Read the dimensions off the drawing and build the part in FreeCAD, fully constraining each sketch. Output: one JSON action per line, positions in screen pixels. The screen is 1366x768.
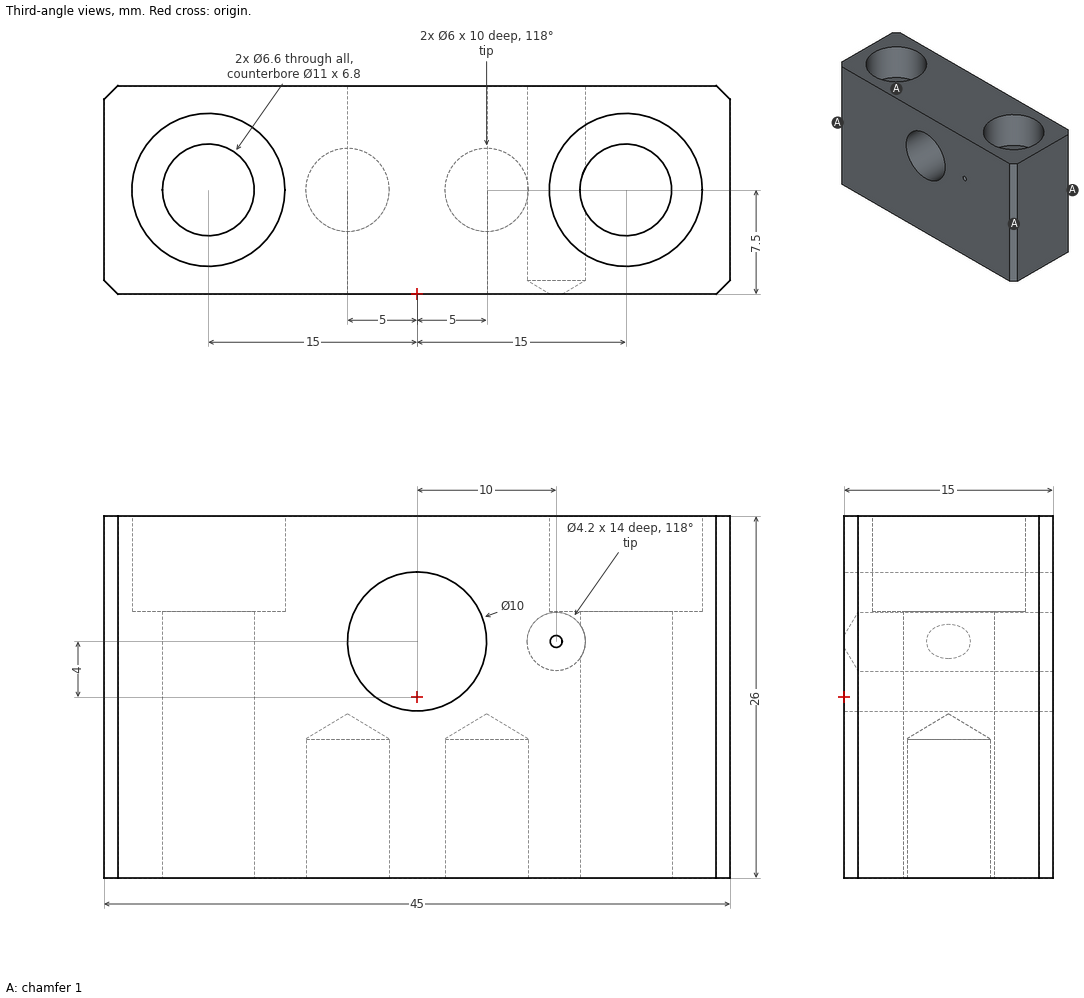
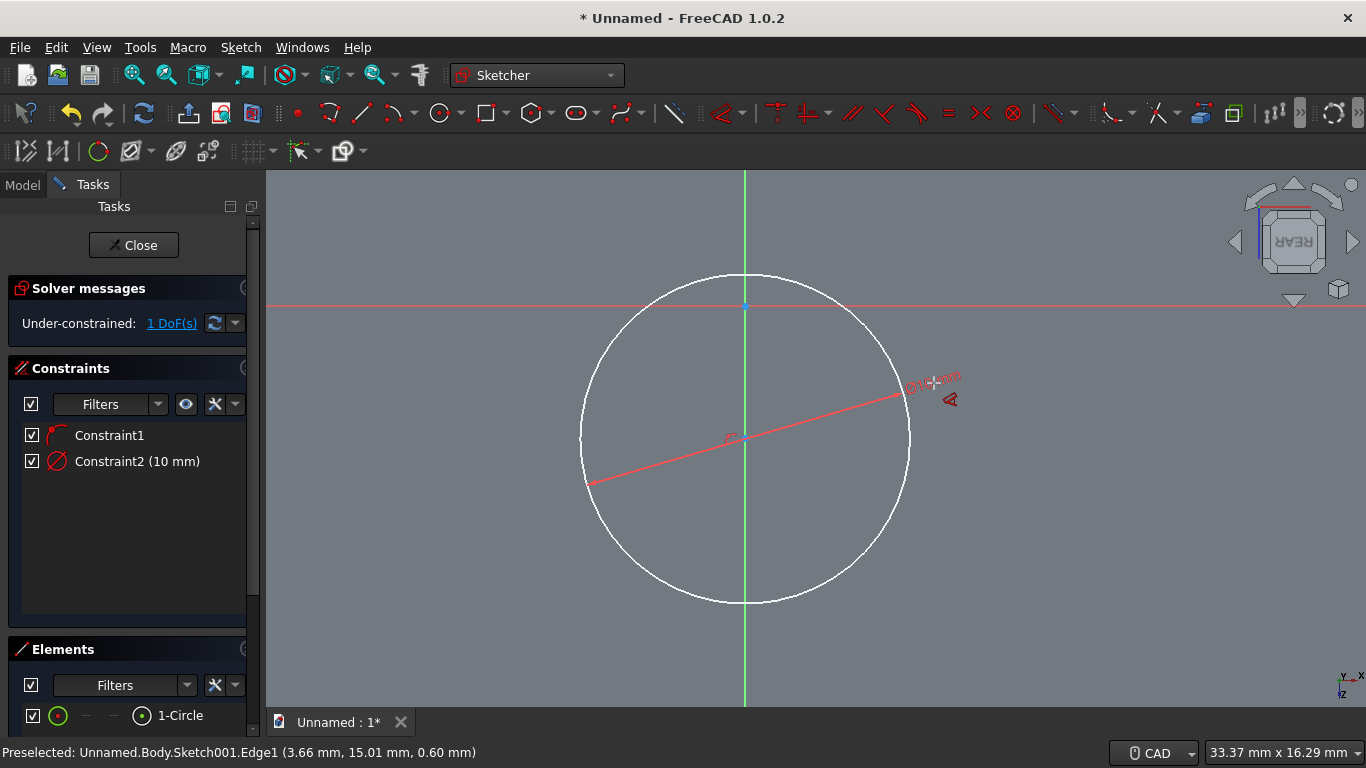
{"action": "left_click", "coordinate": [745, 439]}
{"action": "left_click", "coordinate": [779, 373]}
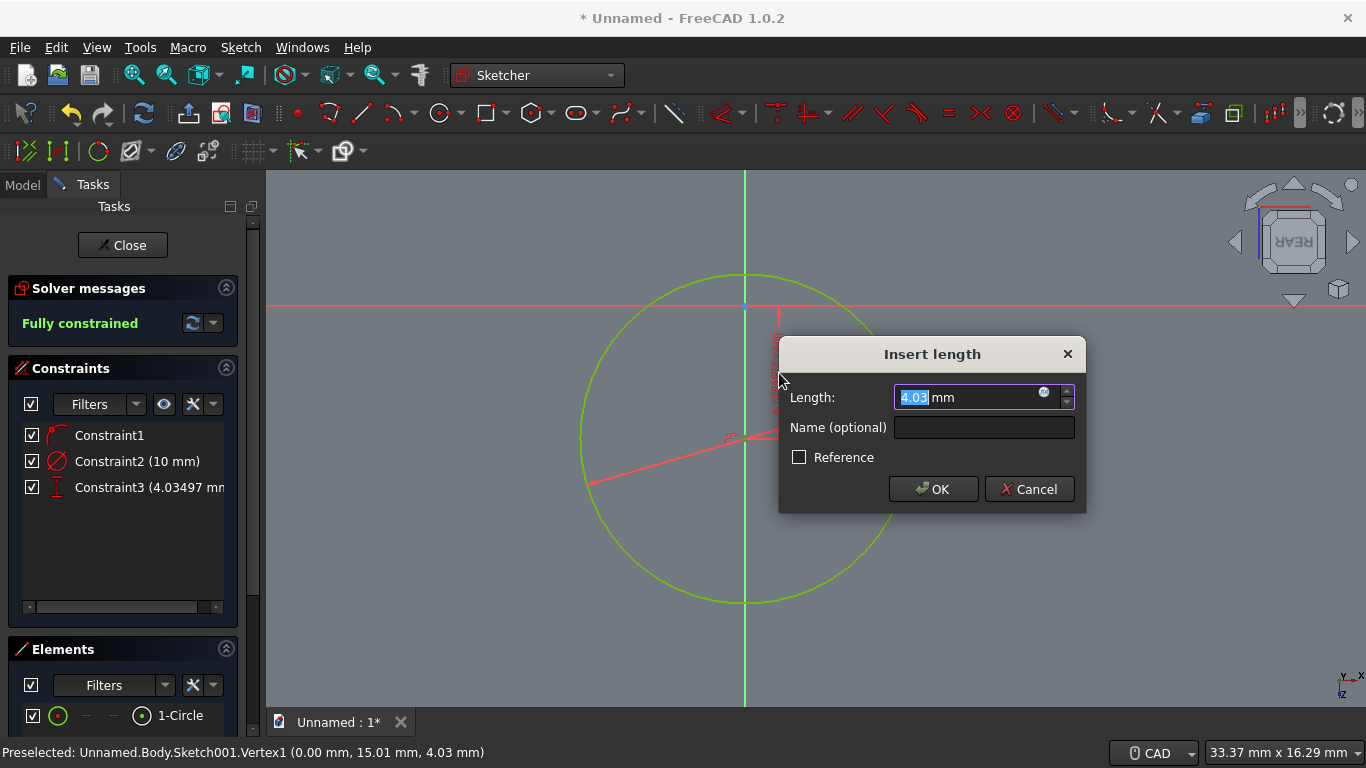
{"action": "type", "text": "4"}
{"action": "key", "text": "Return"}
{"action": "key", "text": "Escape"}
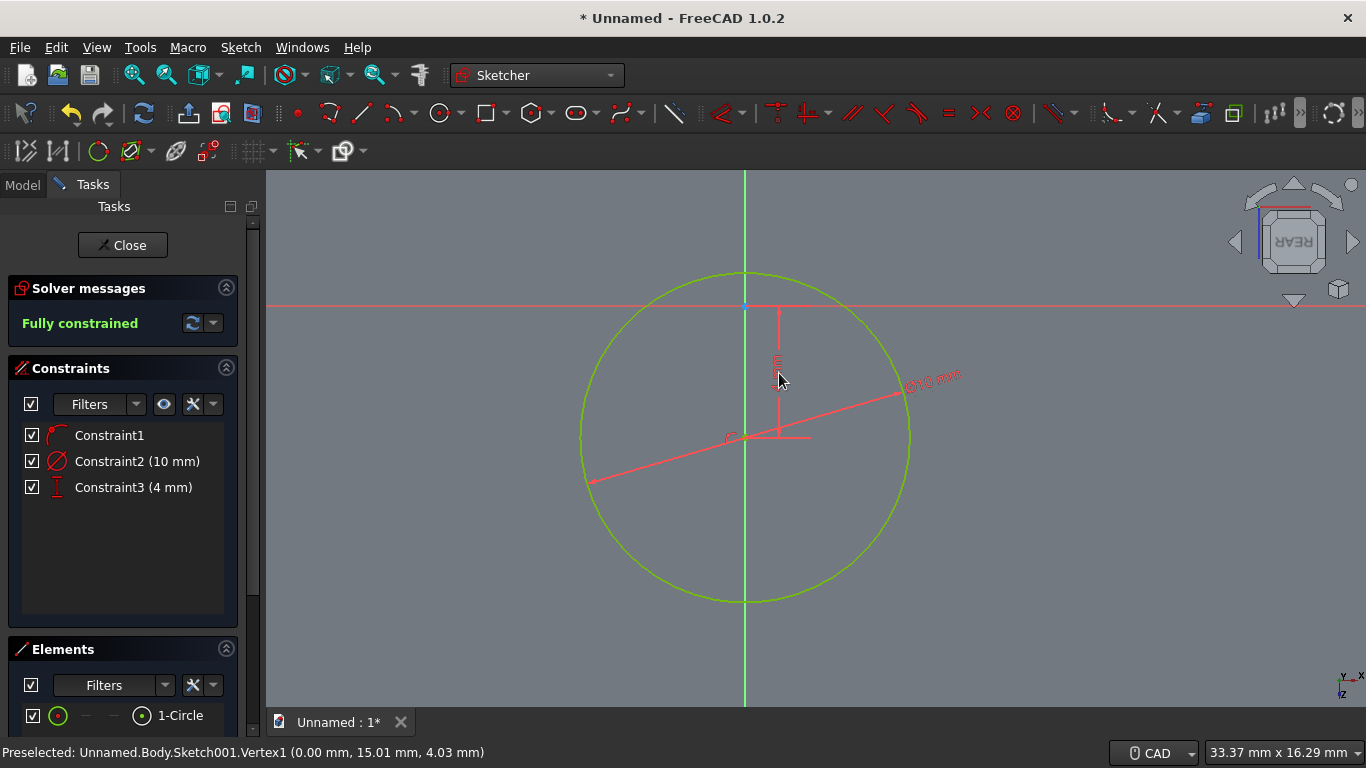
{"action": "left_click", "coordinate": [123, 245]}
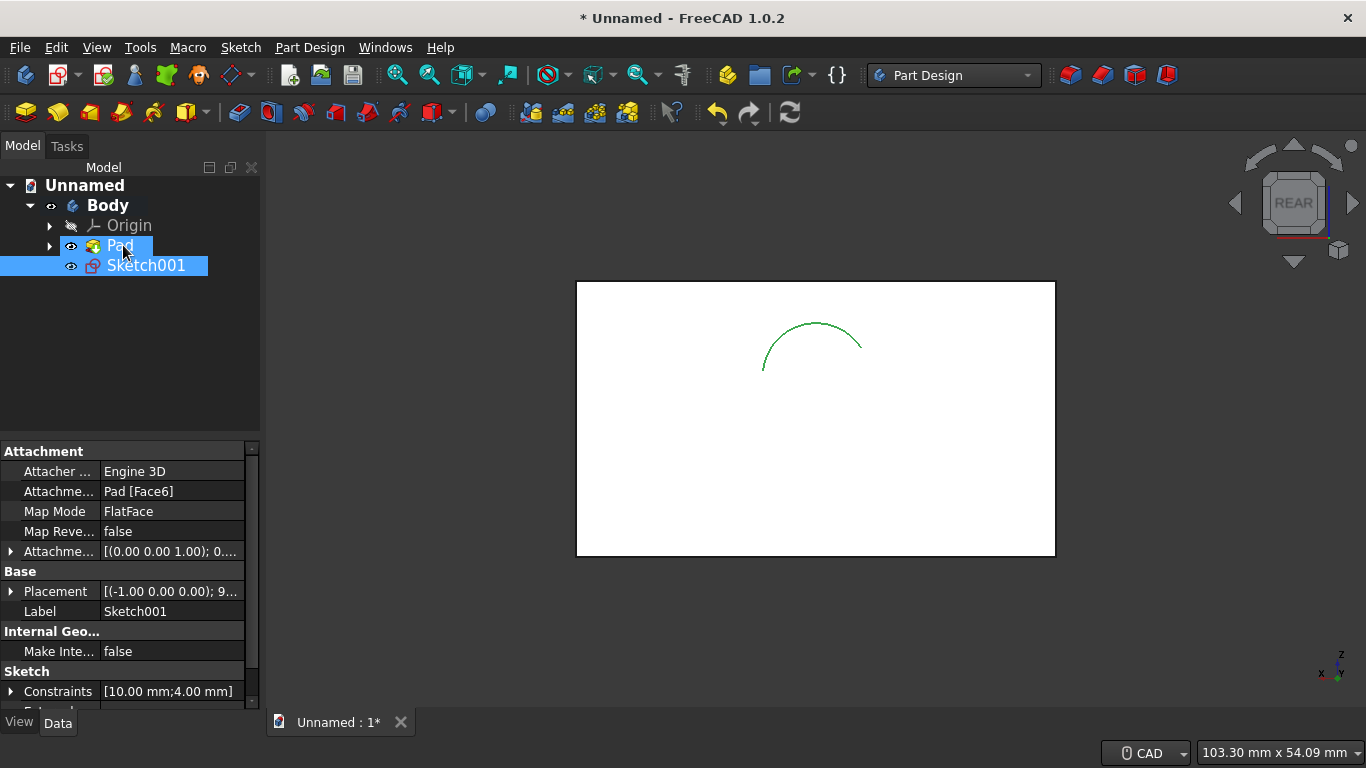
{"action": "left_click", "coordinate": [240, 112]}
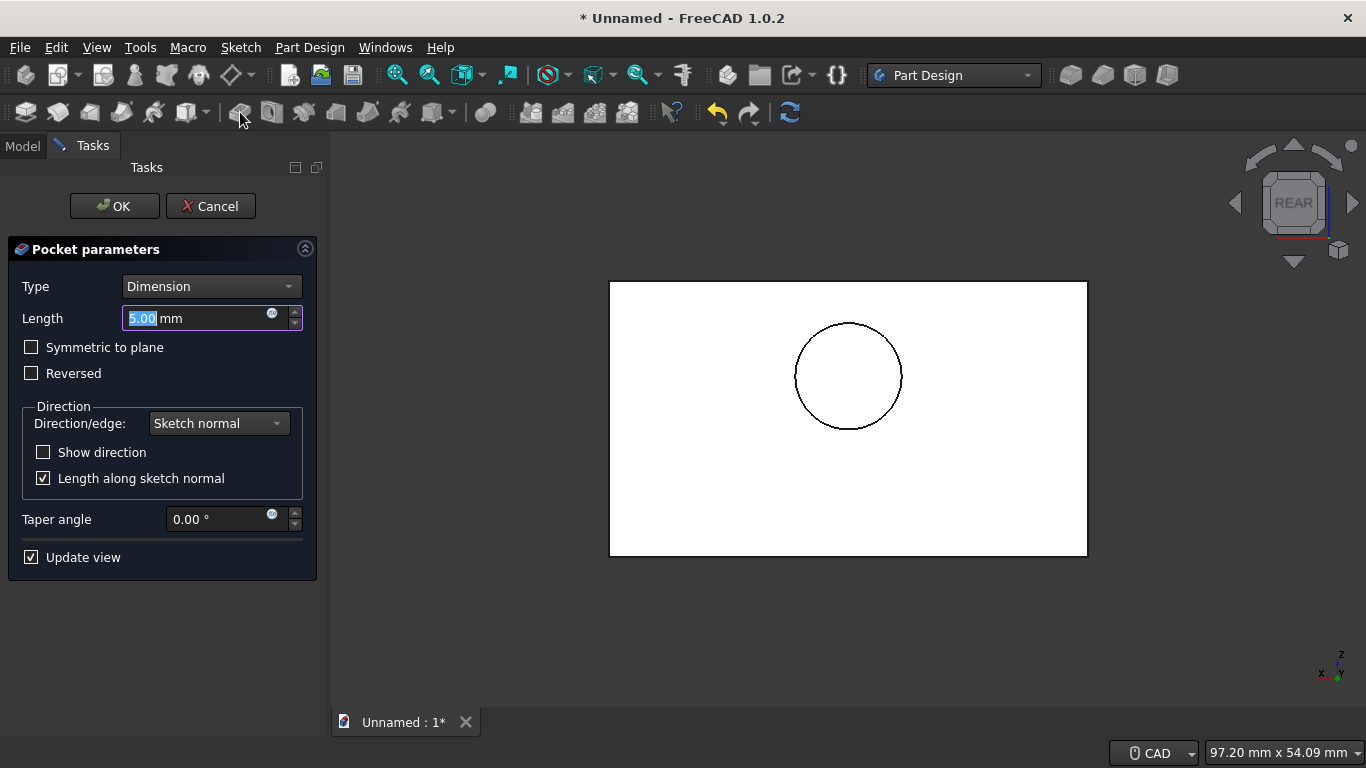
{"action": "left_click", "coordinate": [212, 286]}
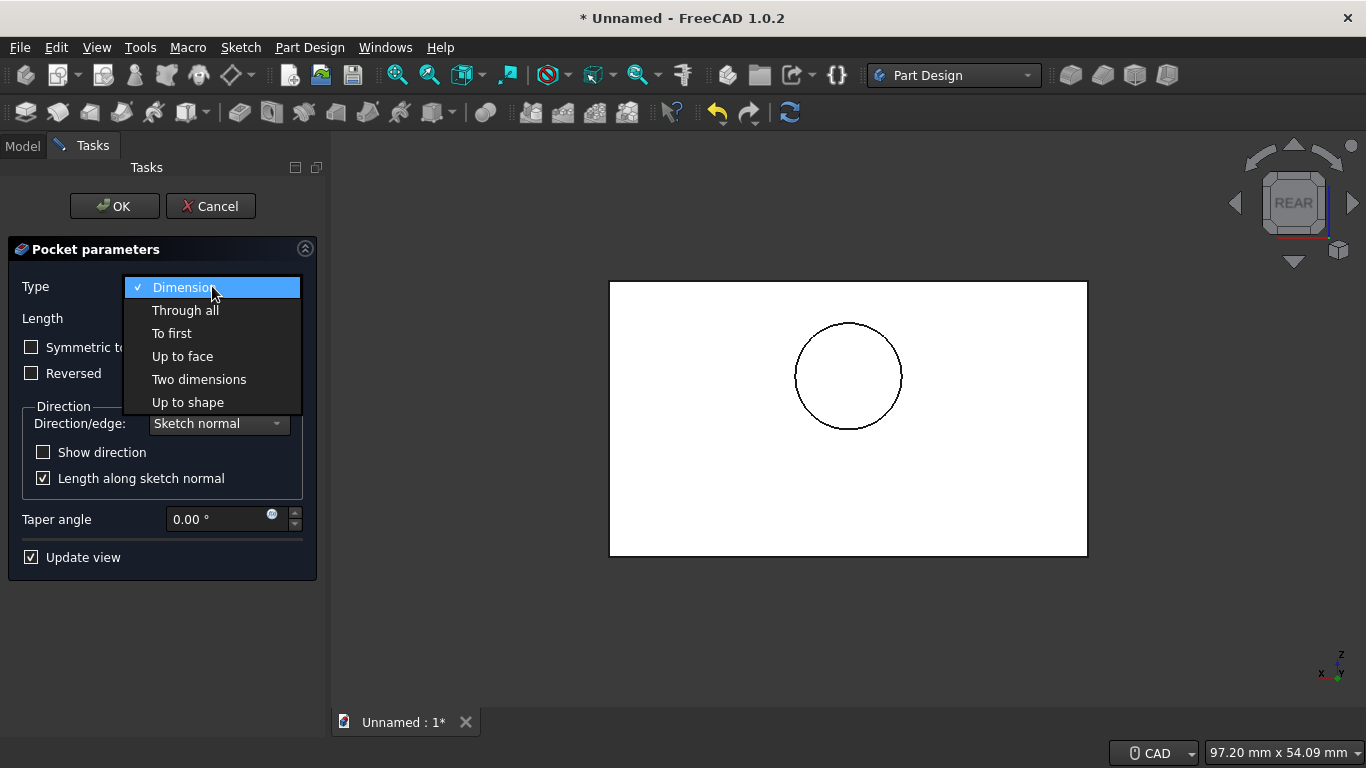
{"action": "left_click", "coordinate": [212, 310]}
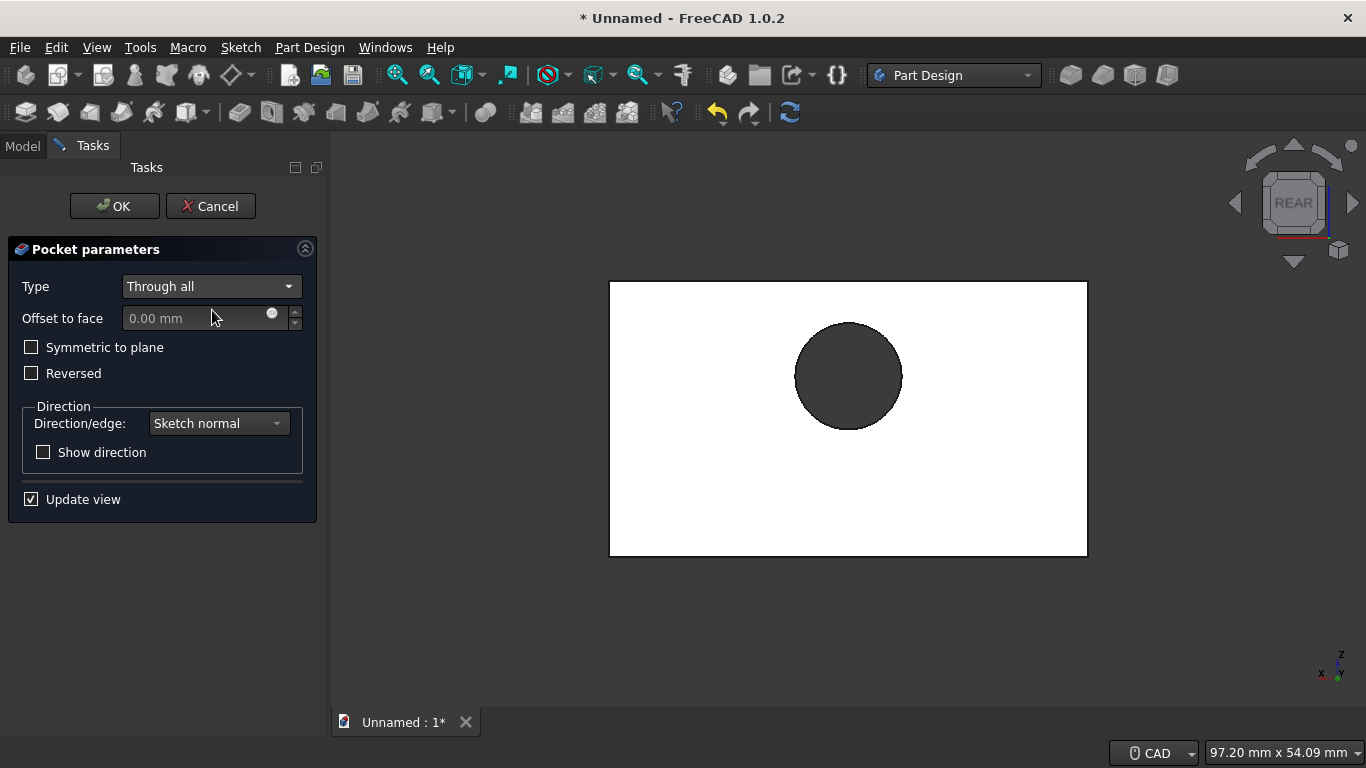
{"action": "left_click", "coordinate": [115, 206]}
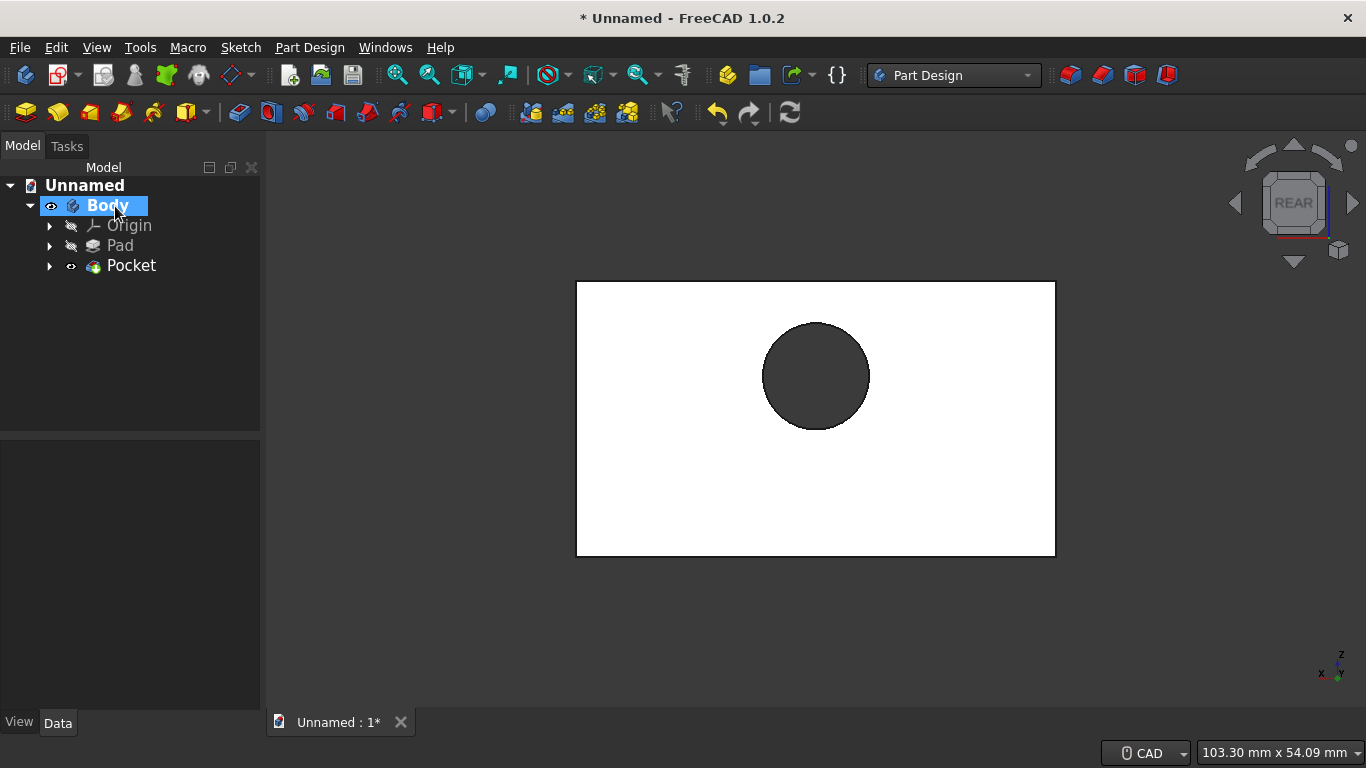
{"action": "key", "text": "5"}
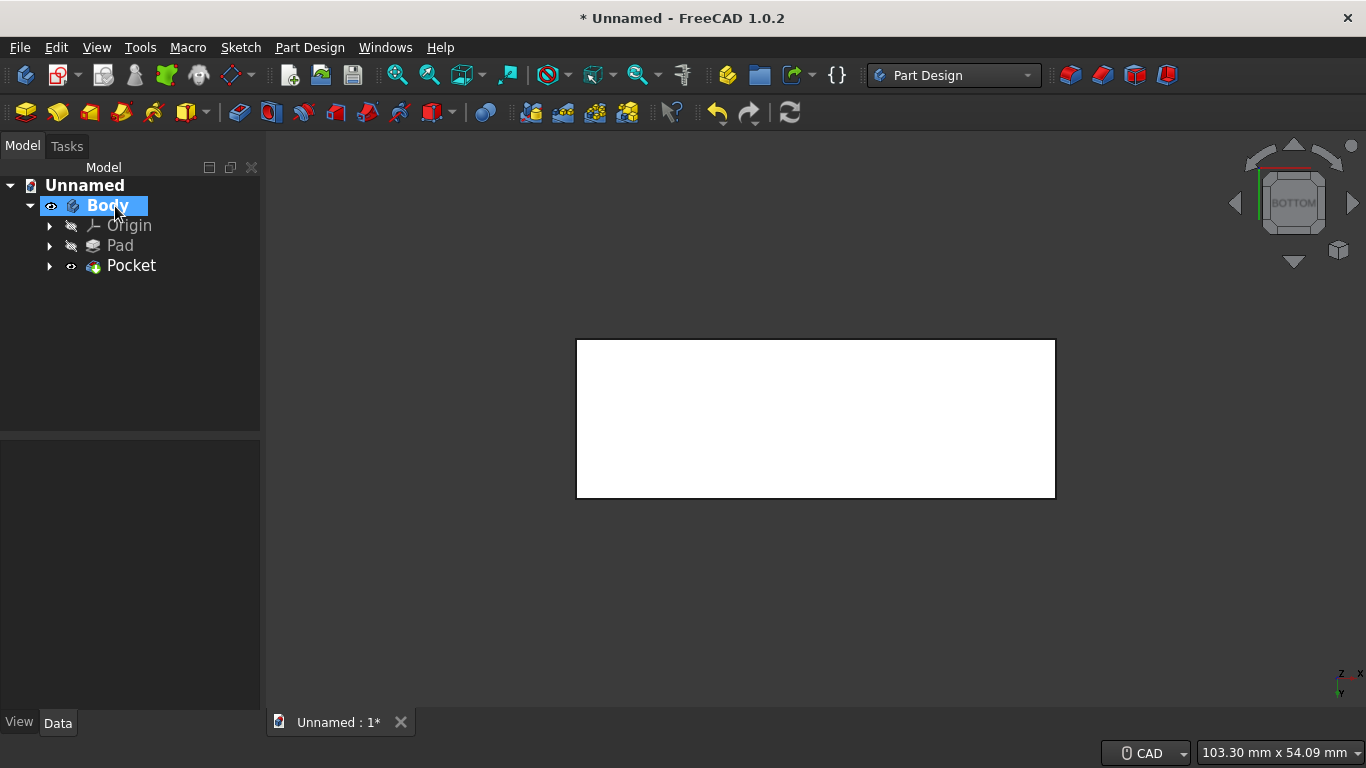
{"action": "left_click", "coordinate": [398, 76]}